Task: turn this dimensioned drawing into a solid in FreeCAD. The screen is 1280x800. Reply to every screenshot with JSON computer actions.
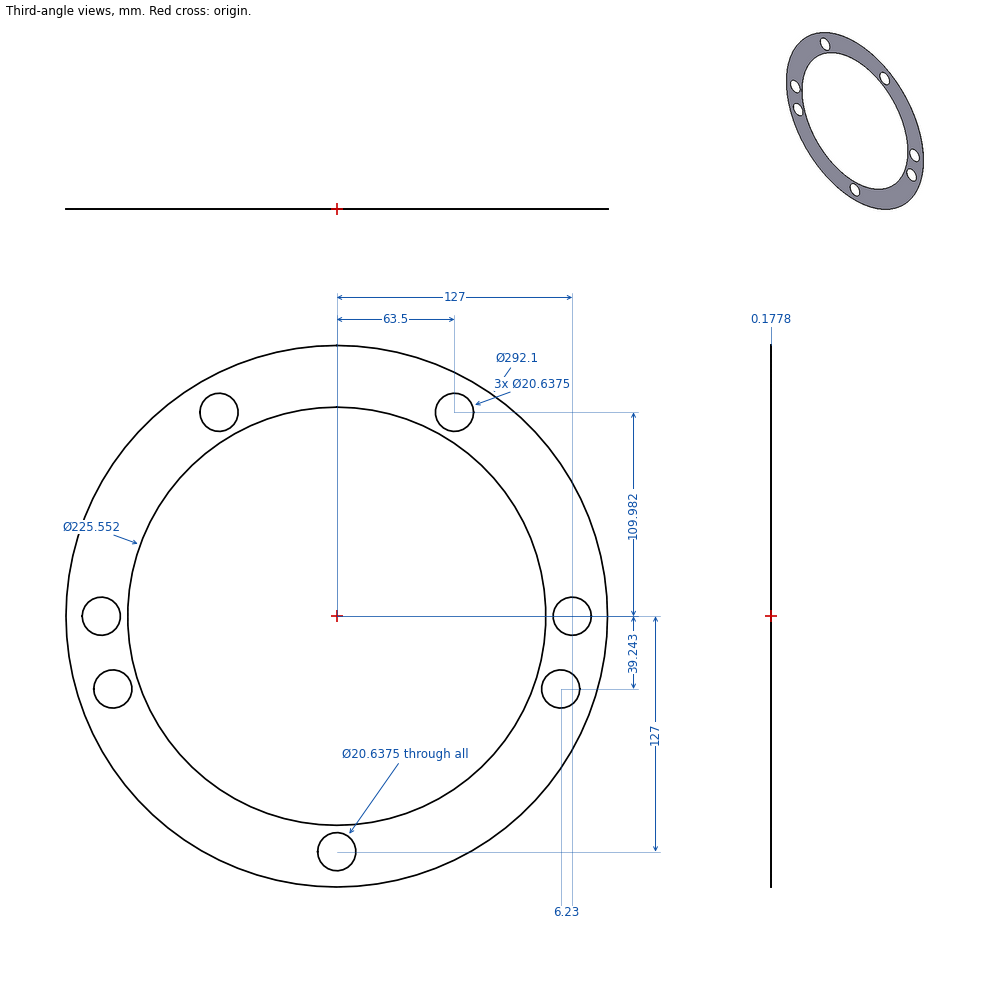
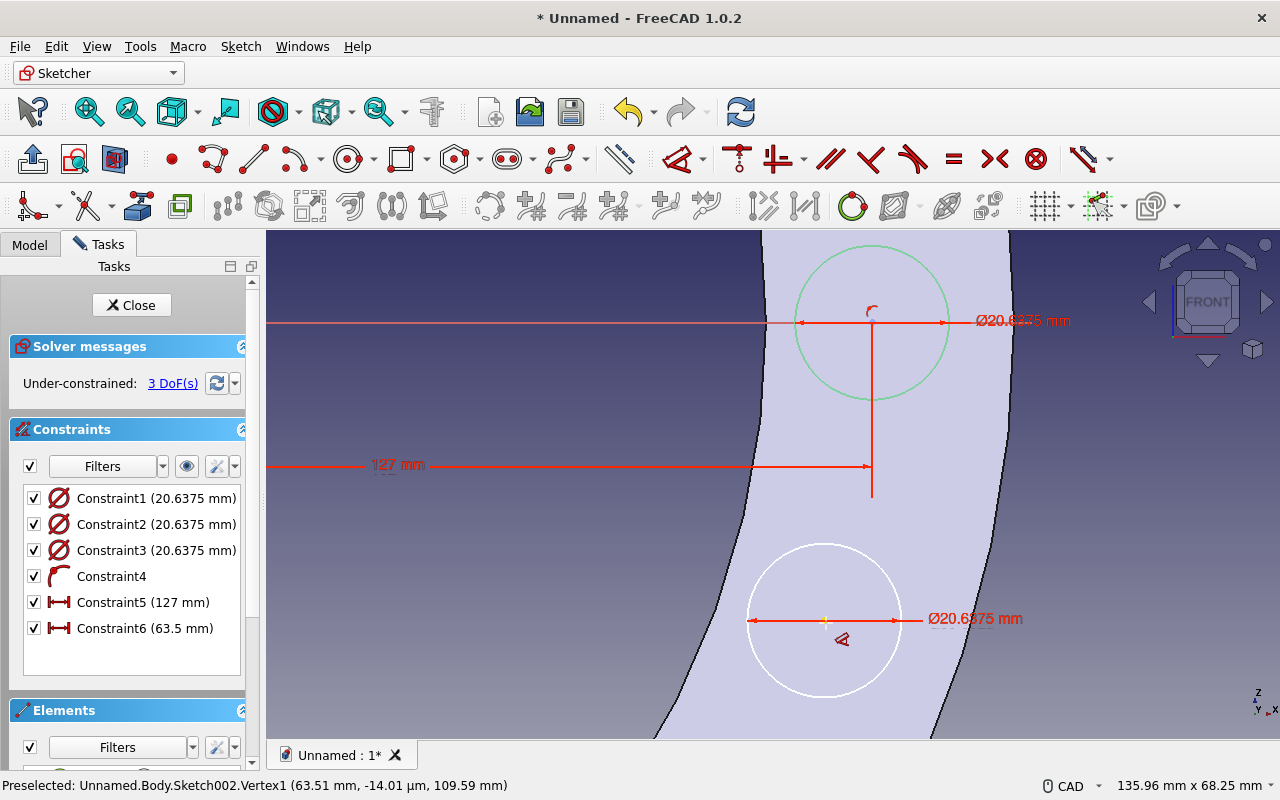
{"action": "left_click", "coordinate": [824, 621]}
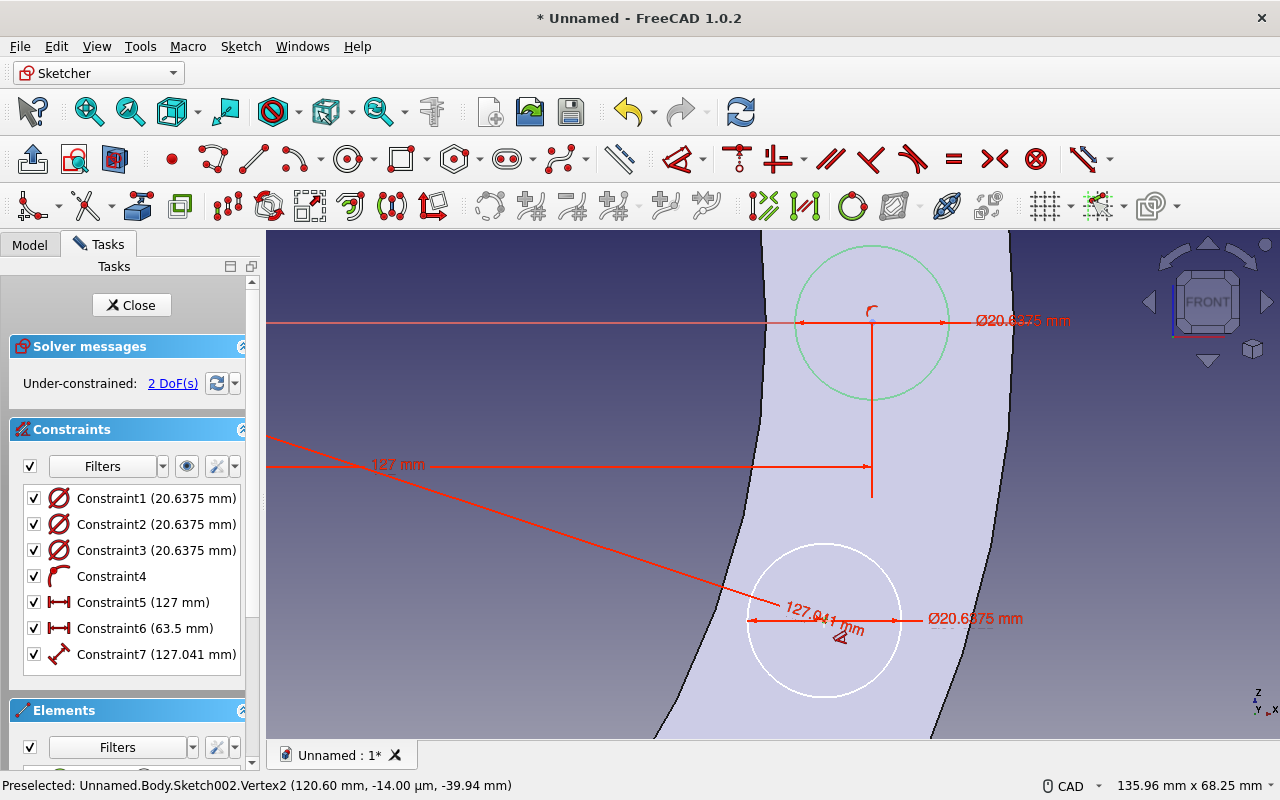
{"action": "left_click", "coordinate": [872, 323]}
{"action": "left_click", "coordinate": [848, 655]}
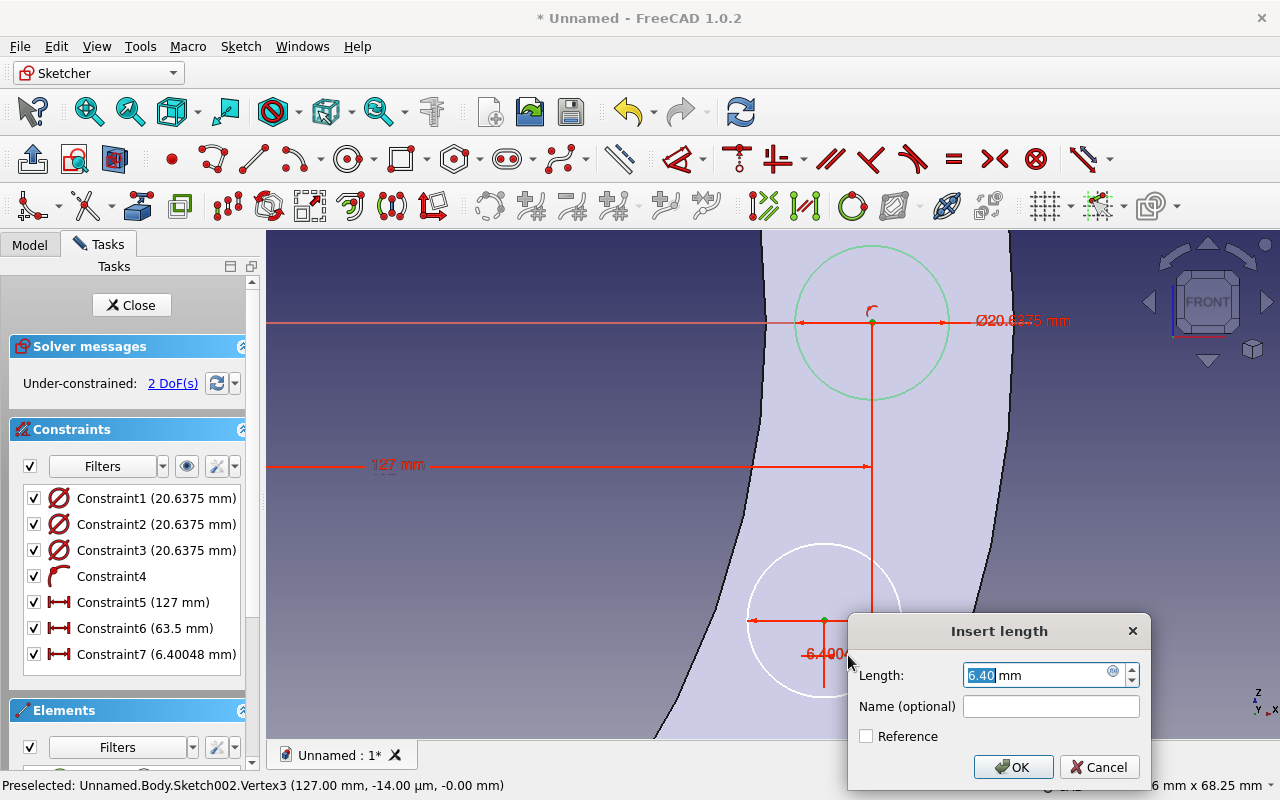
{"action": "type", "text": "6.23"}
{"action": "key", "text": "Return"}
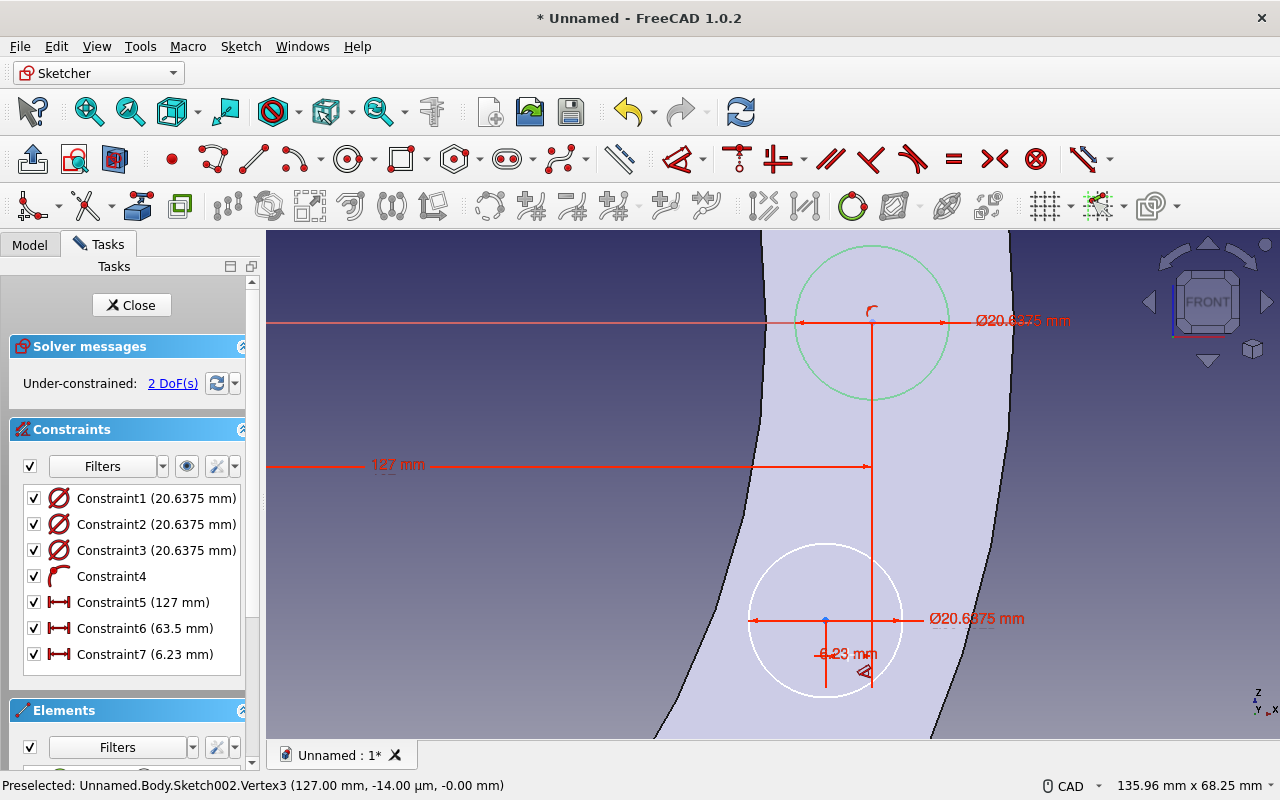
{"action": "scroll", "coordinate": [792, 624], "scroll_direction": "down", "scroll_amount": 7}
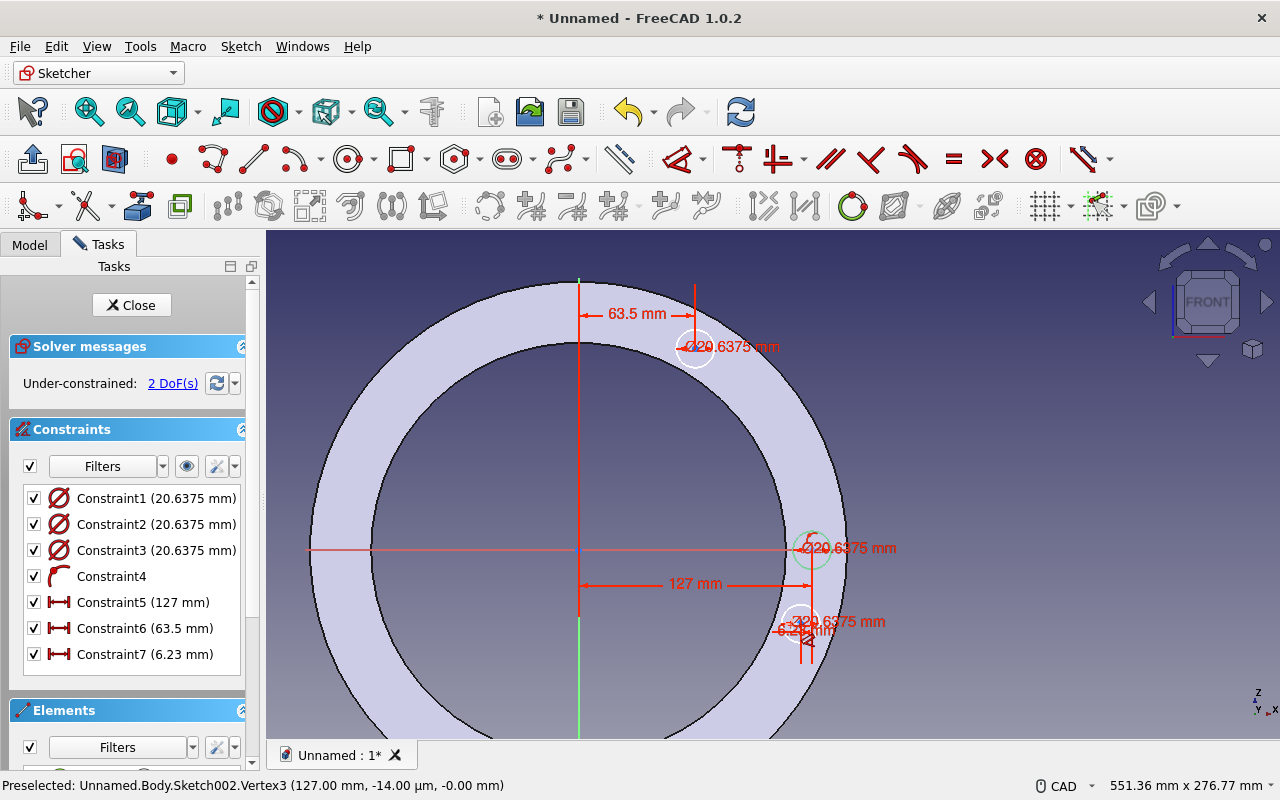
{"action": "left_click", "coordinate": [801, 624]}
{"action": "left_click", "coordinate": [545, 587]}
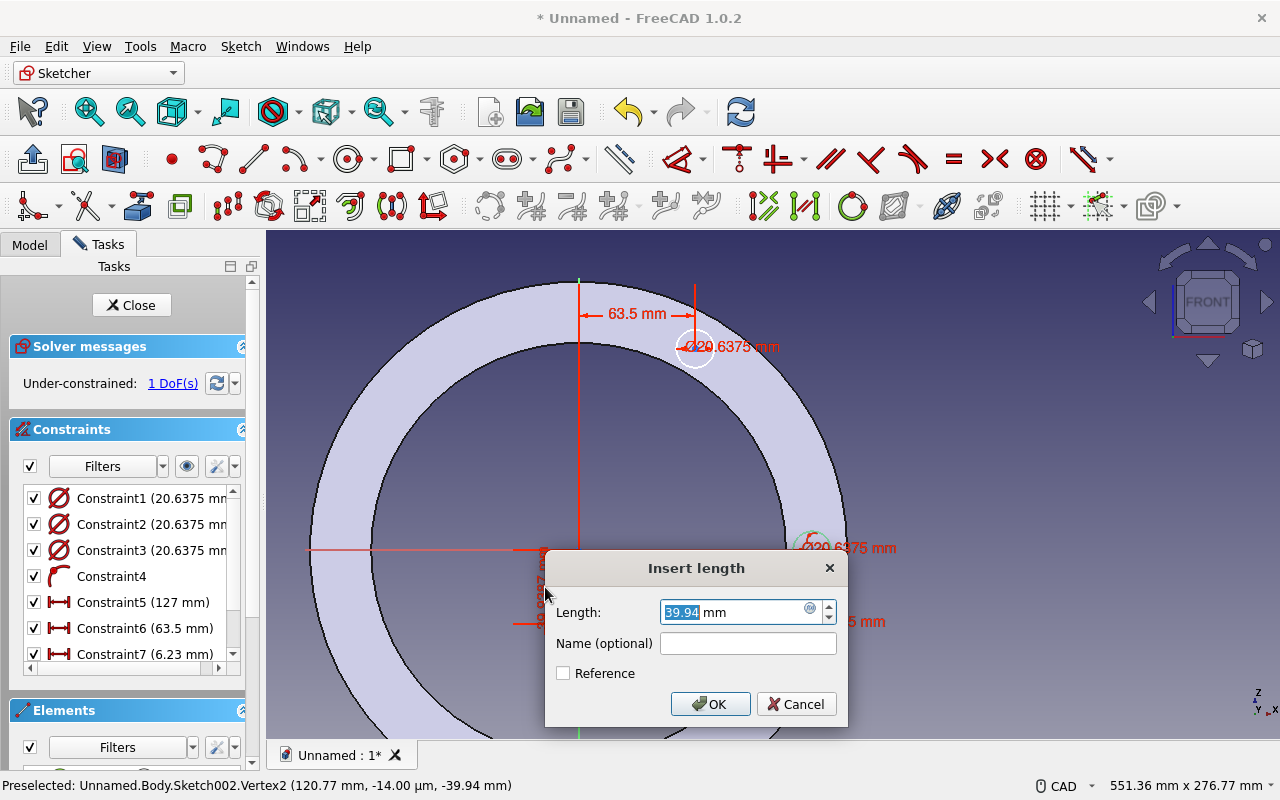
{"action": "type", "text": "39.243"}
{"action": "key", "text": "Return"}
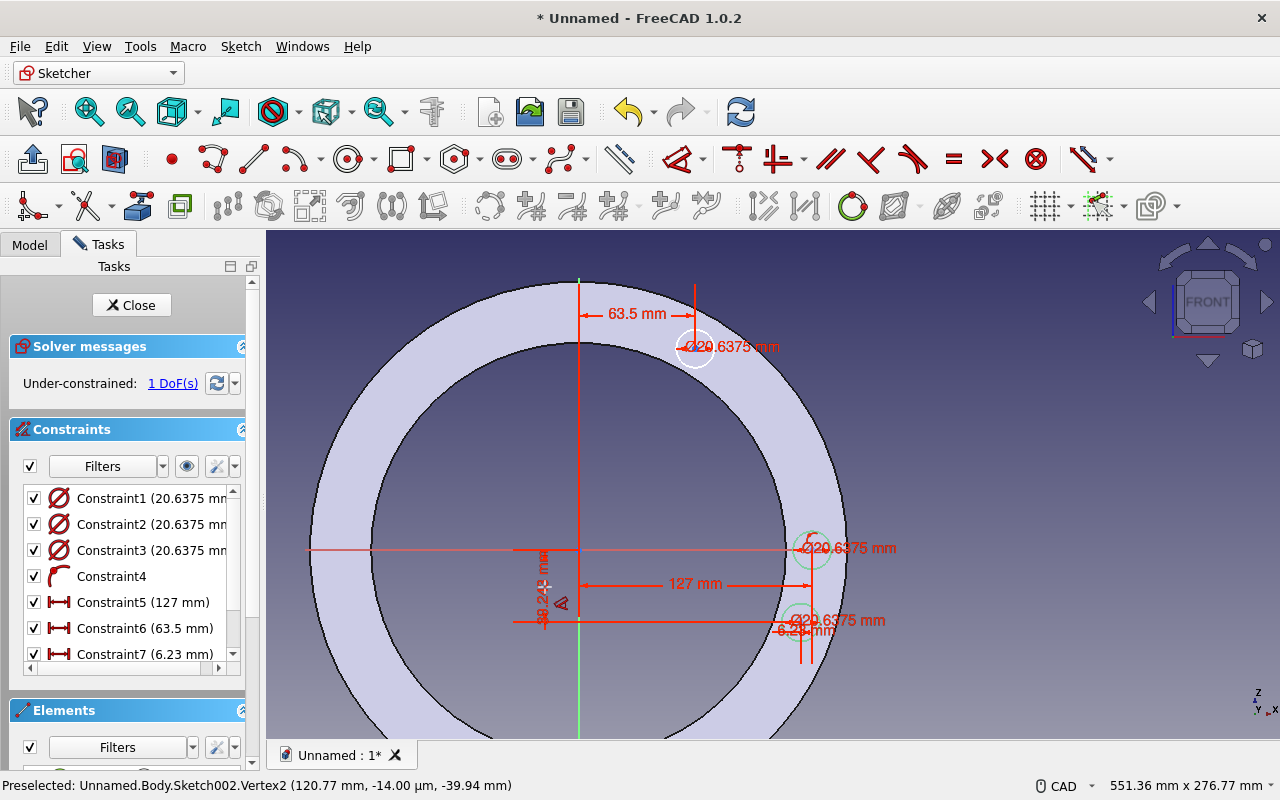
{"action": "left_click", "coordinate": [695, 349]}
{"action": "left_click", "coordinate": [545, 450]}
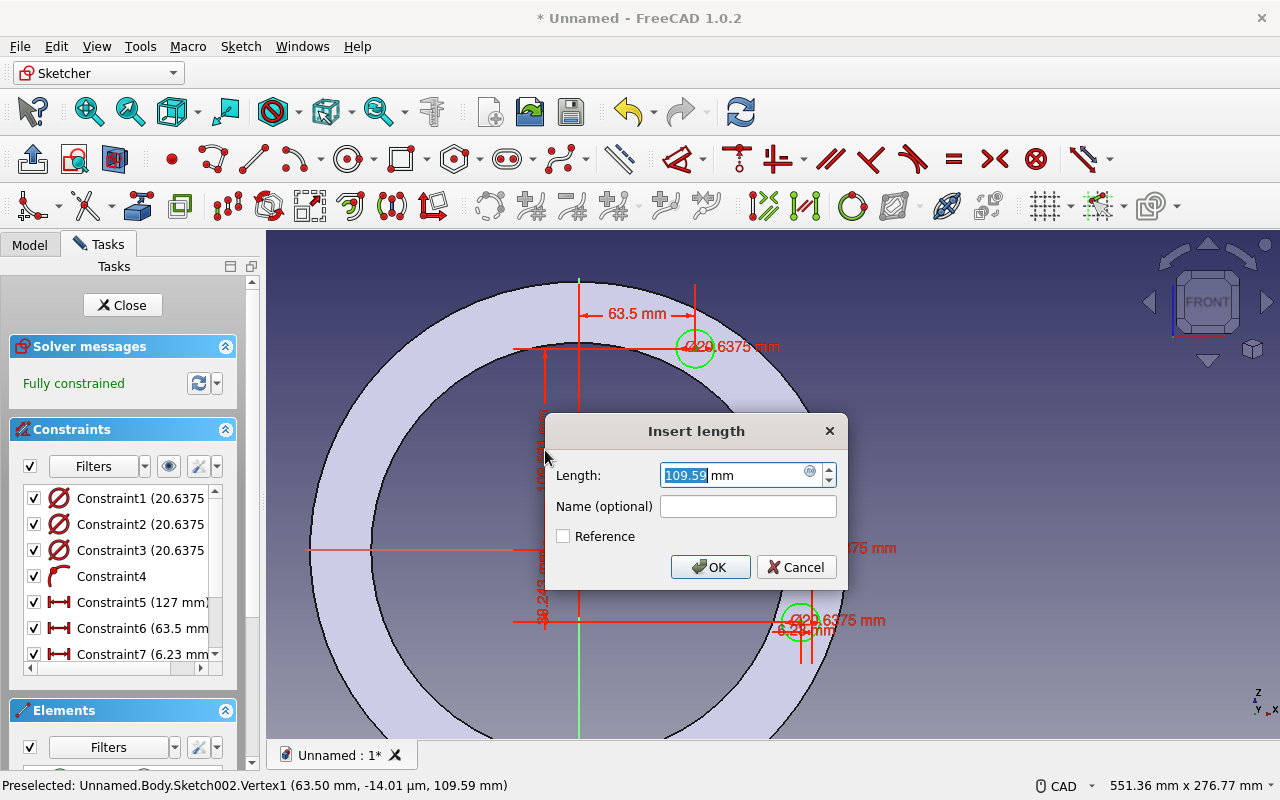
{"action": "type", "text": "109.982"}
{"action": "key", "text": "Return"}
{"action": "key", "text": "Escape"}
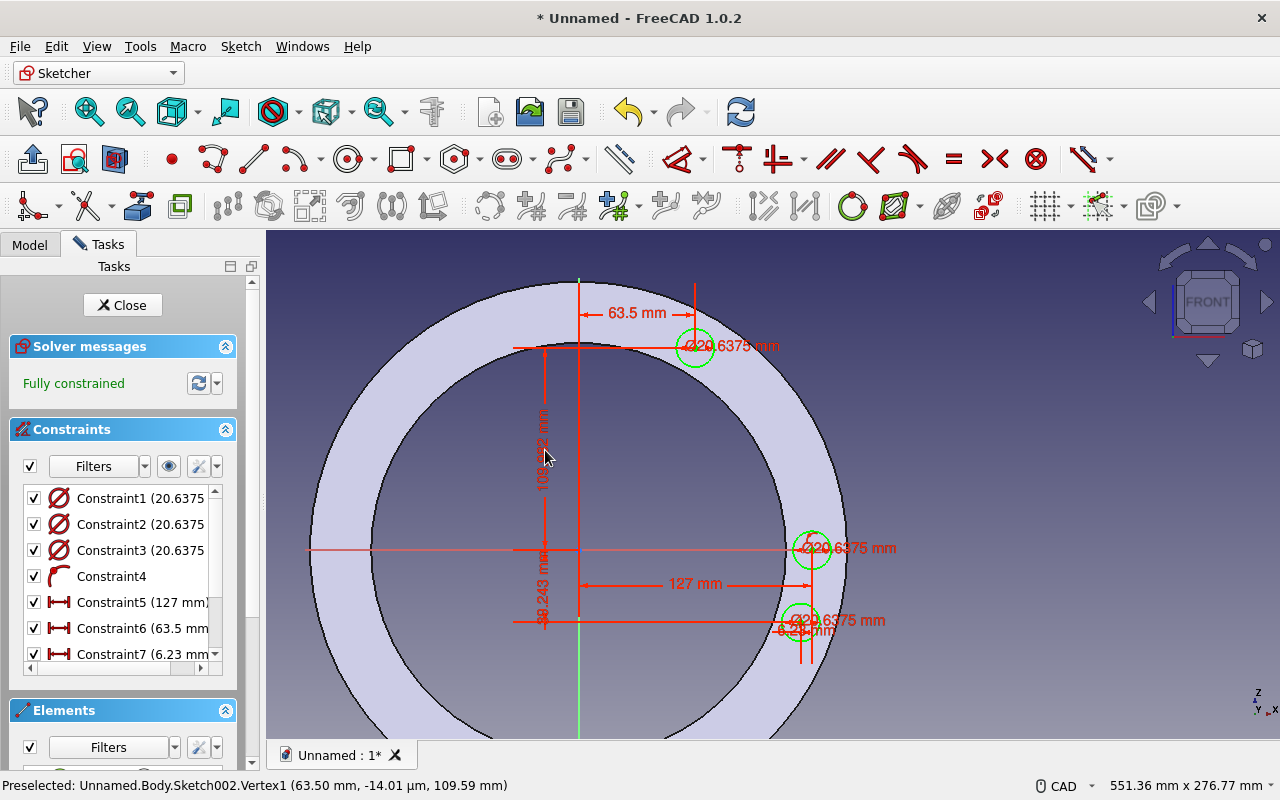
{"action": "left_click", "coordinate": [123, 305]}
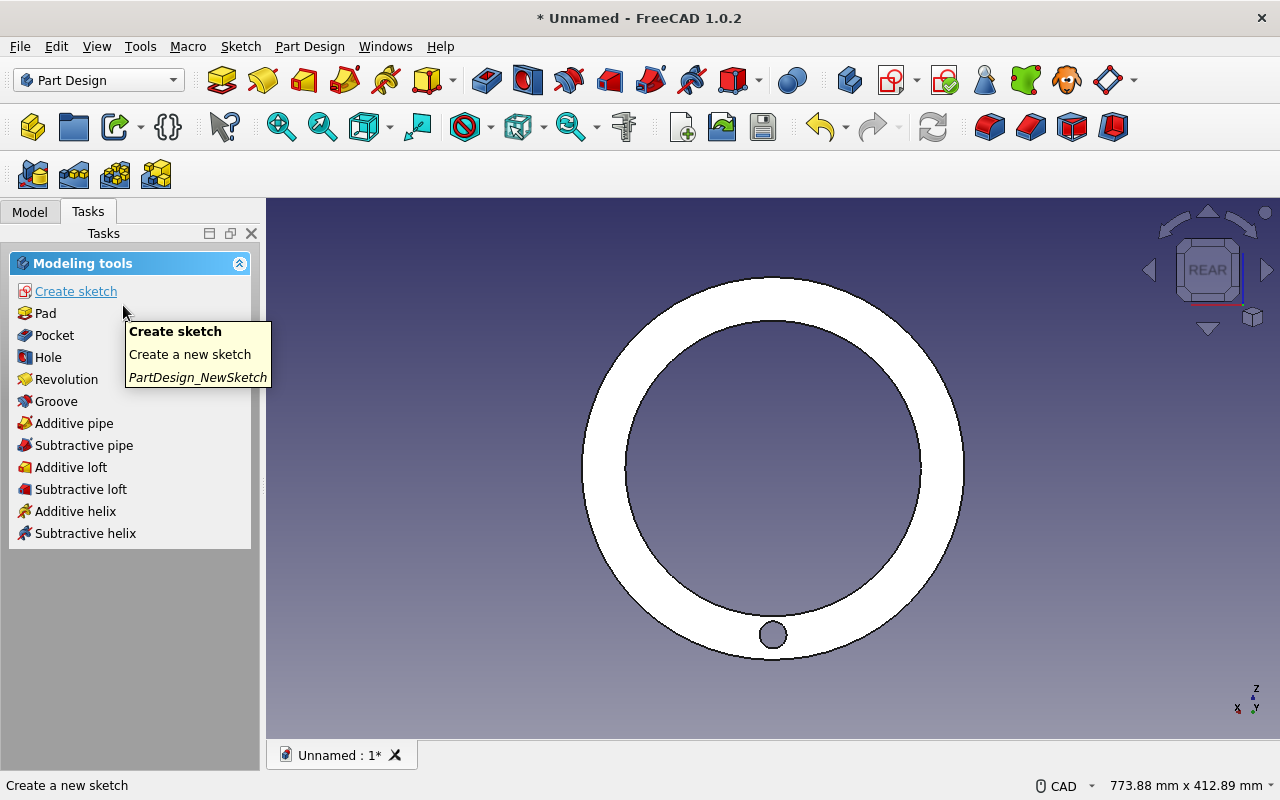
{"action": "left_click", "coordinate": [487, 80]}